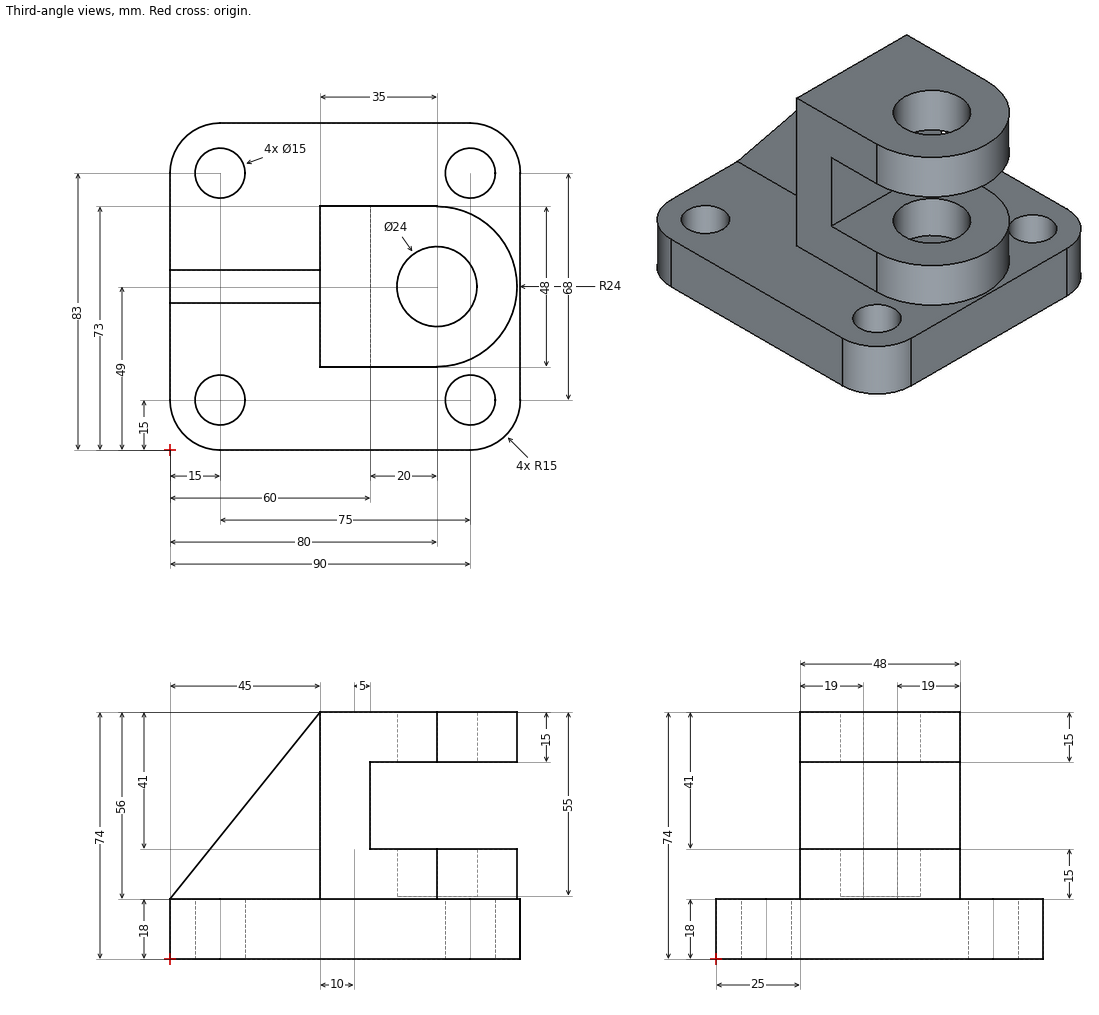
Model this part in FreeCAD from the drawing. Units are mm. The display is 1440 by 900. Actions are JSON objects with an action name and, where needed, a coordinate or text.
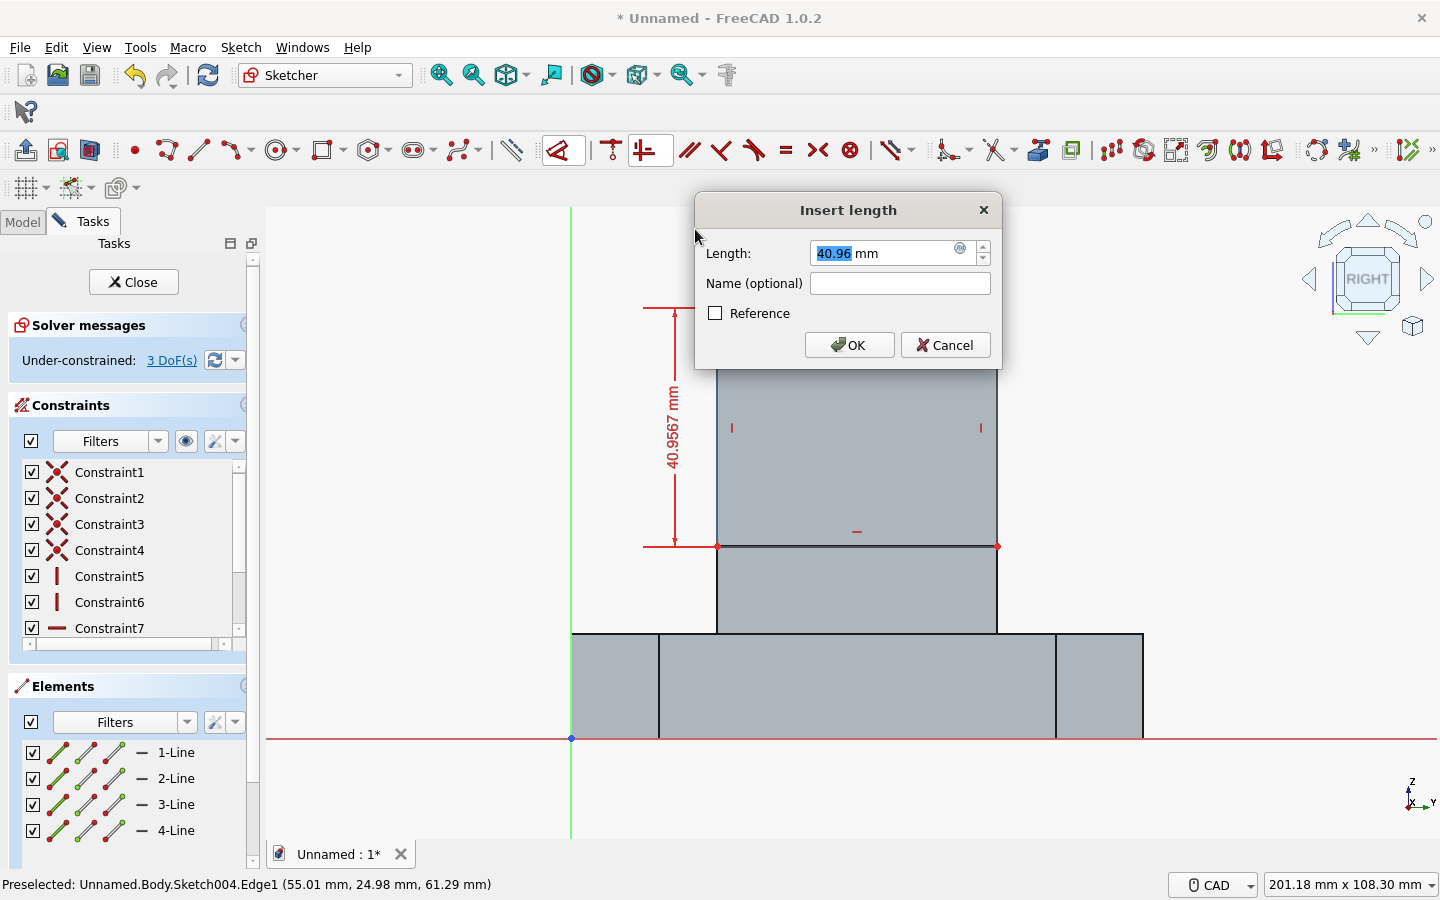
{"action": "type", "text": "41"}
{"action": "key", "text": "Return"}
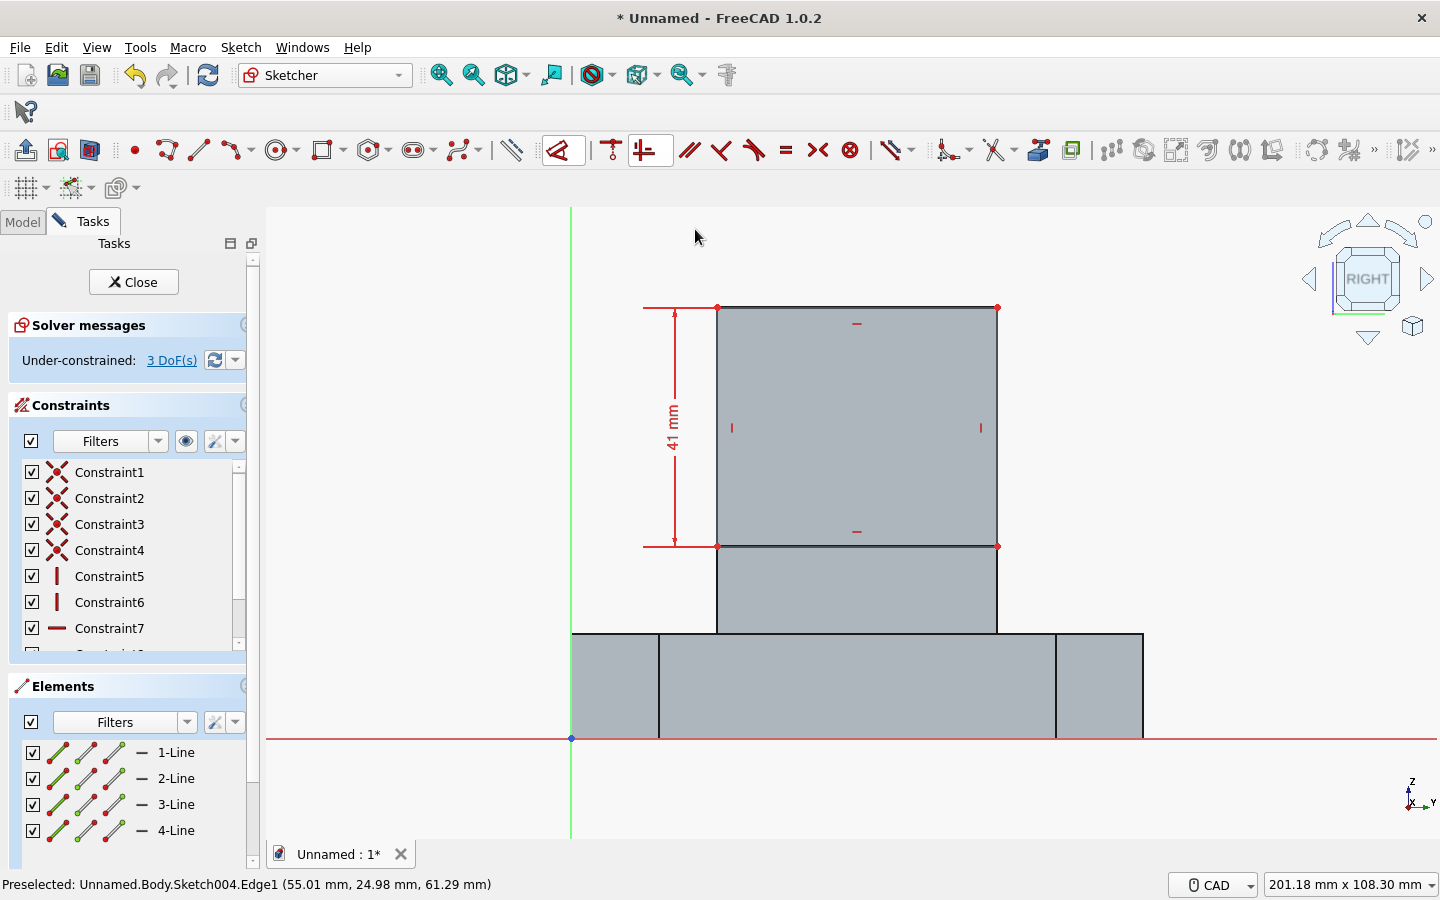
{"action": "left_click", "coordinate": [801, 547]}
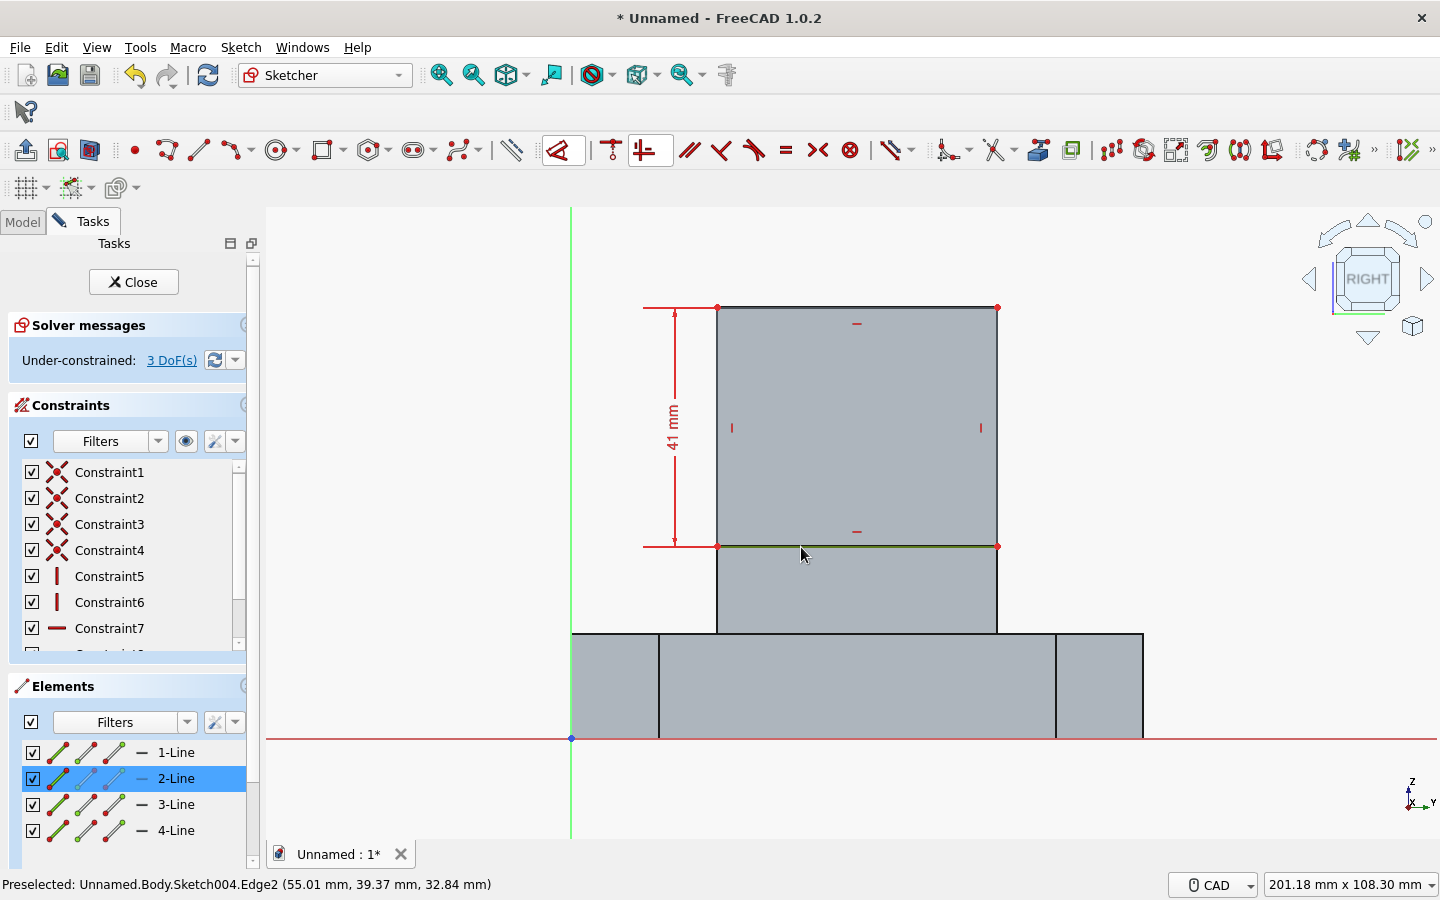
{"action": "left_click", "coordinate": [580, 150]}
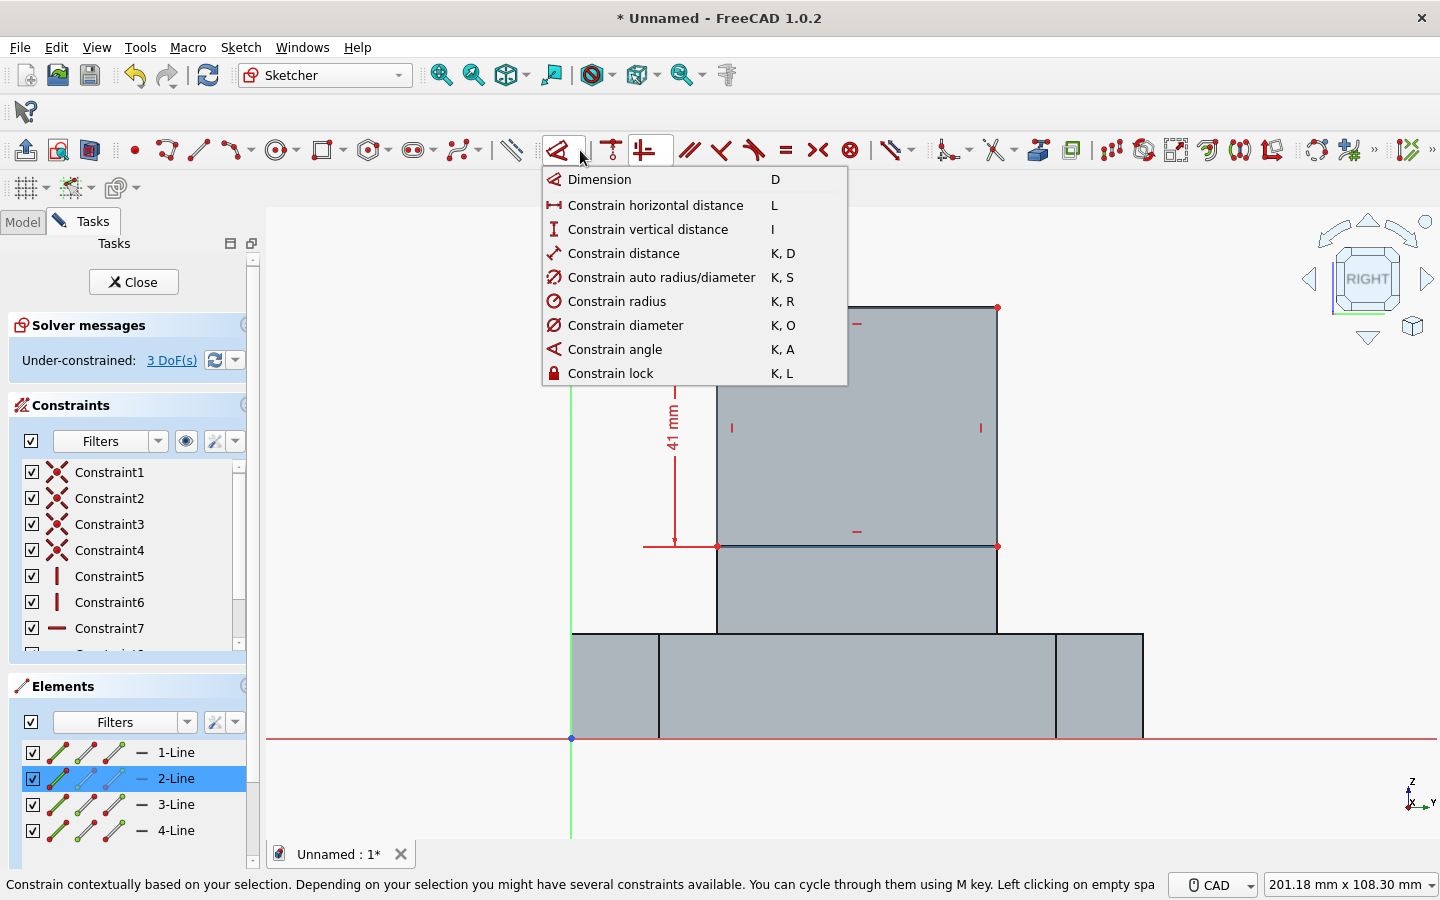
{"action": "left_click", "coordinate": [695, 205]}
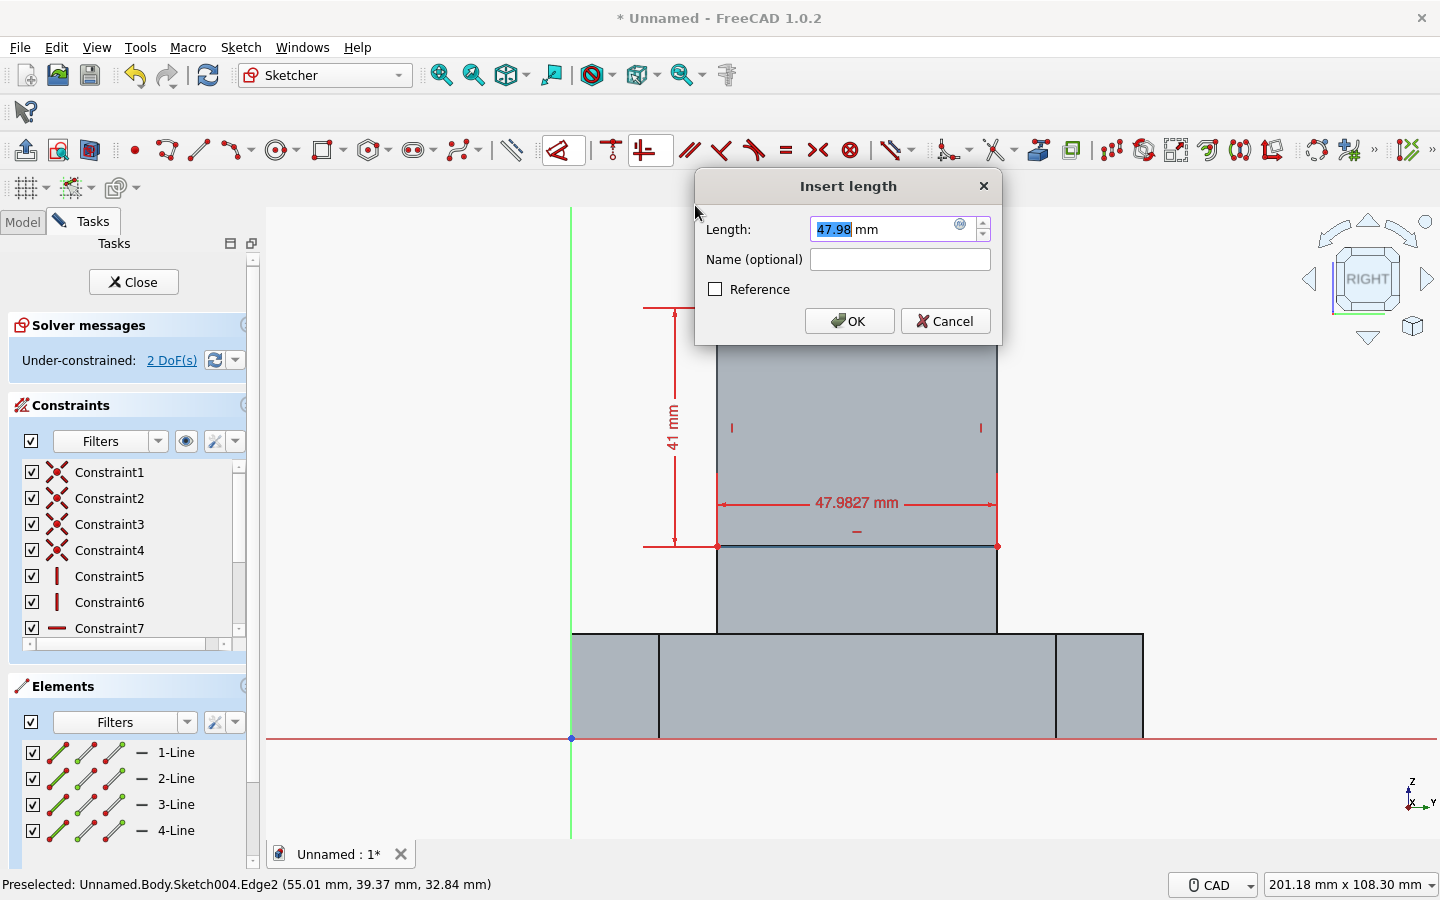
{"action": "type", "text": "48"}
{"action": "key", "text": "Return"}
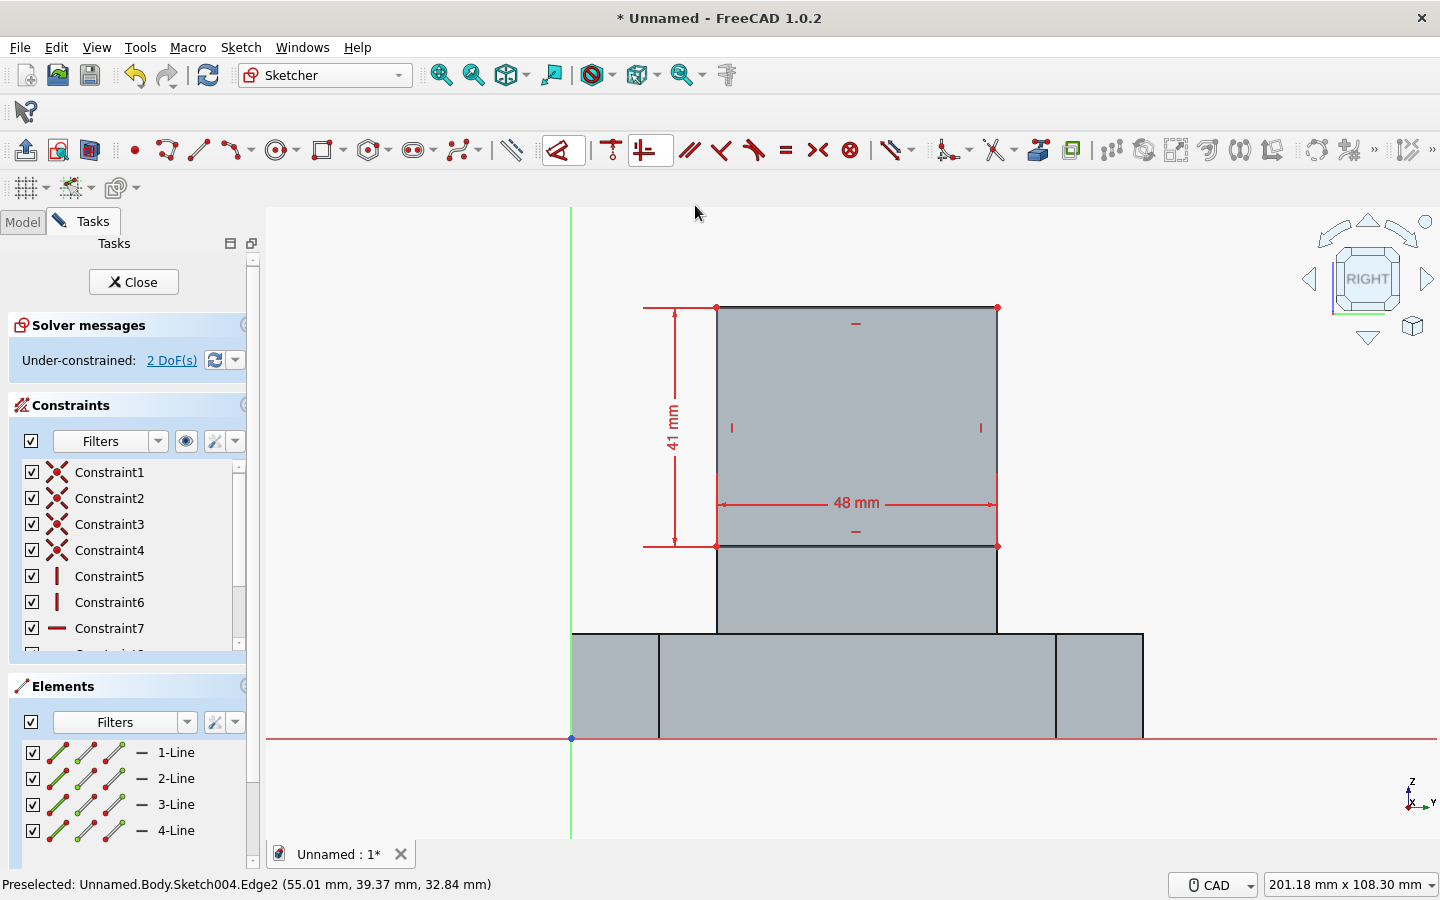
{"action": "left_click", "coordinate": [717, 308]}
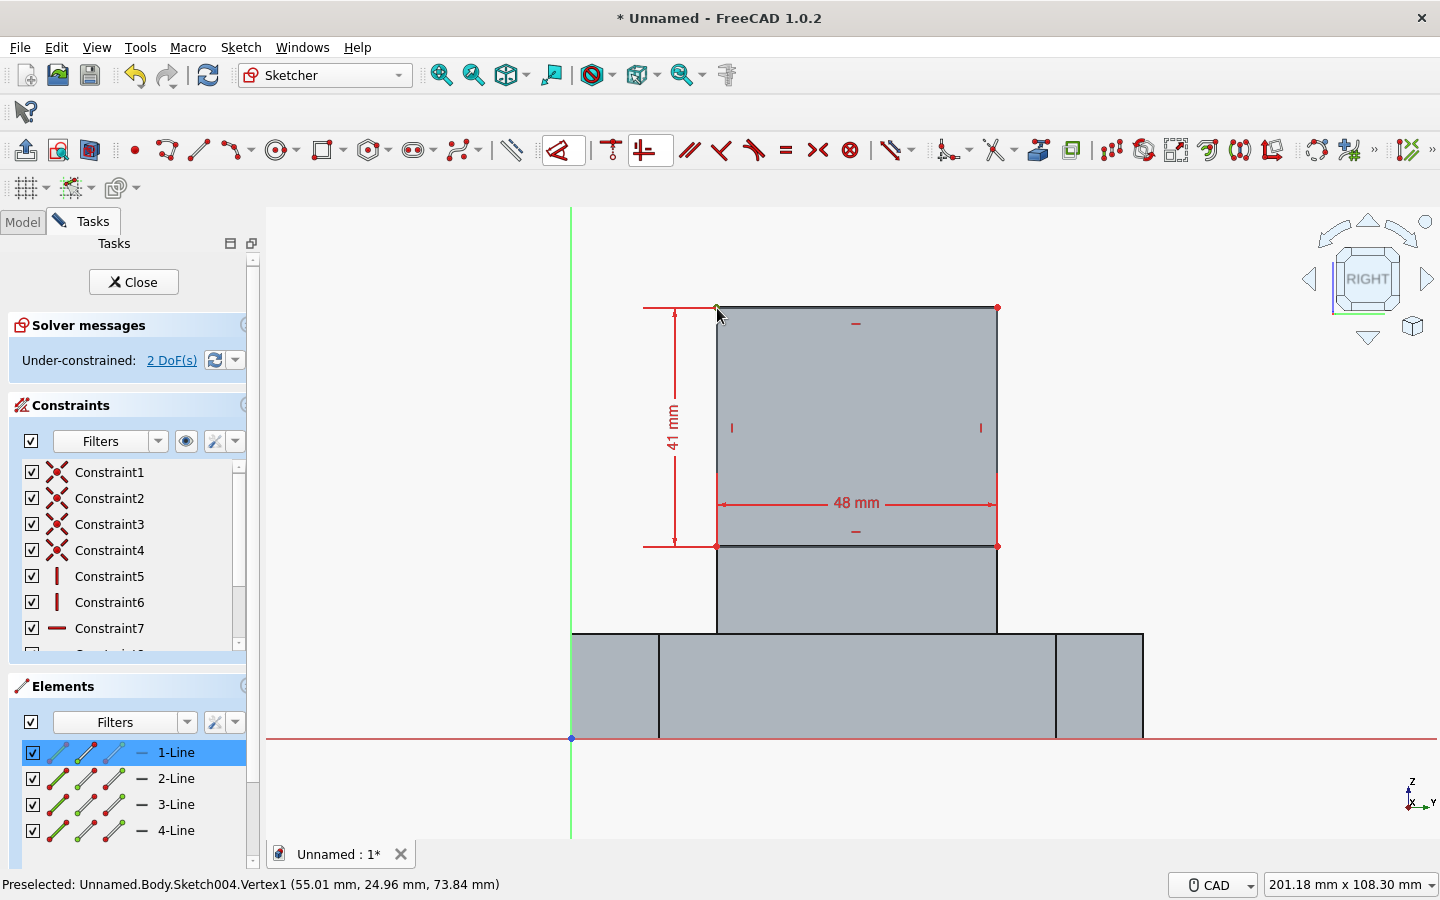
{"action": "key", "text": "l"}